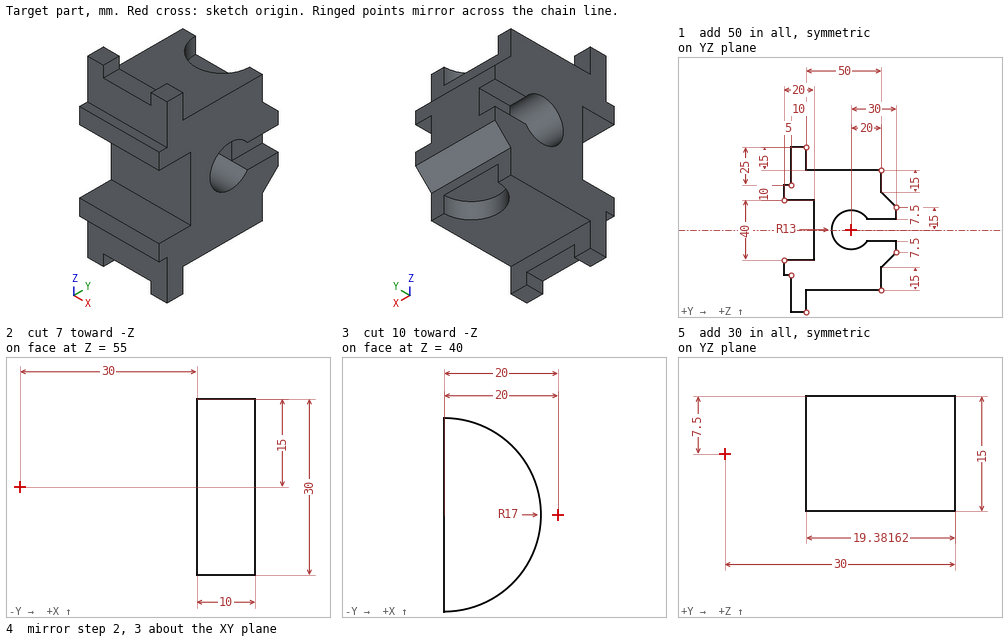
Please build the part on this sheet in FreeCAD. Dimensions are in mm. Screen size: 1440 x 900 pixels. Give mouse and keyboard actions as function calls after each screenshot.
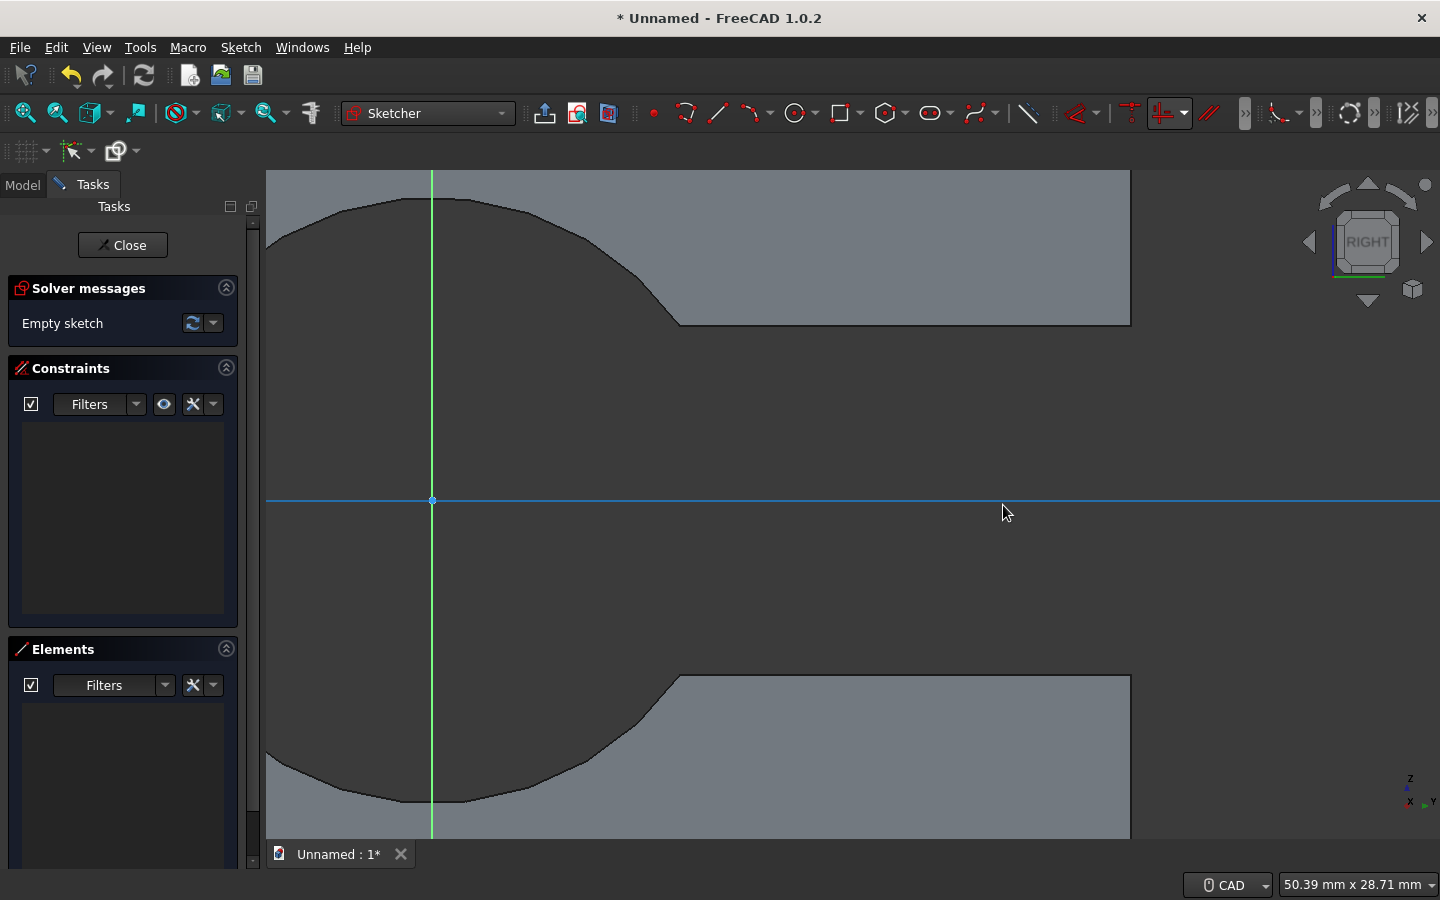
click(840, 114)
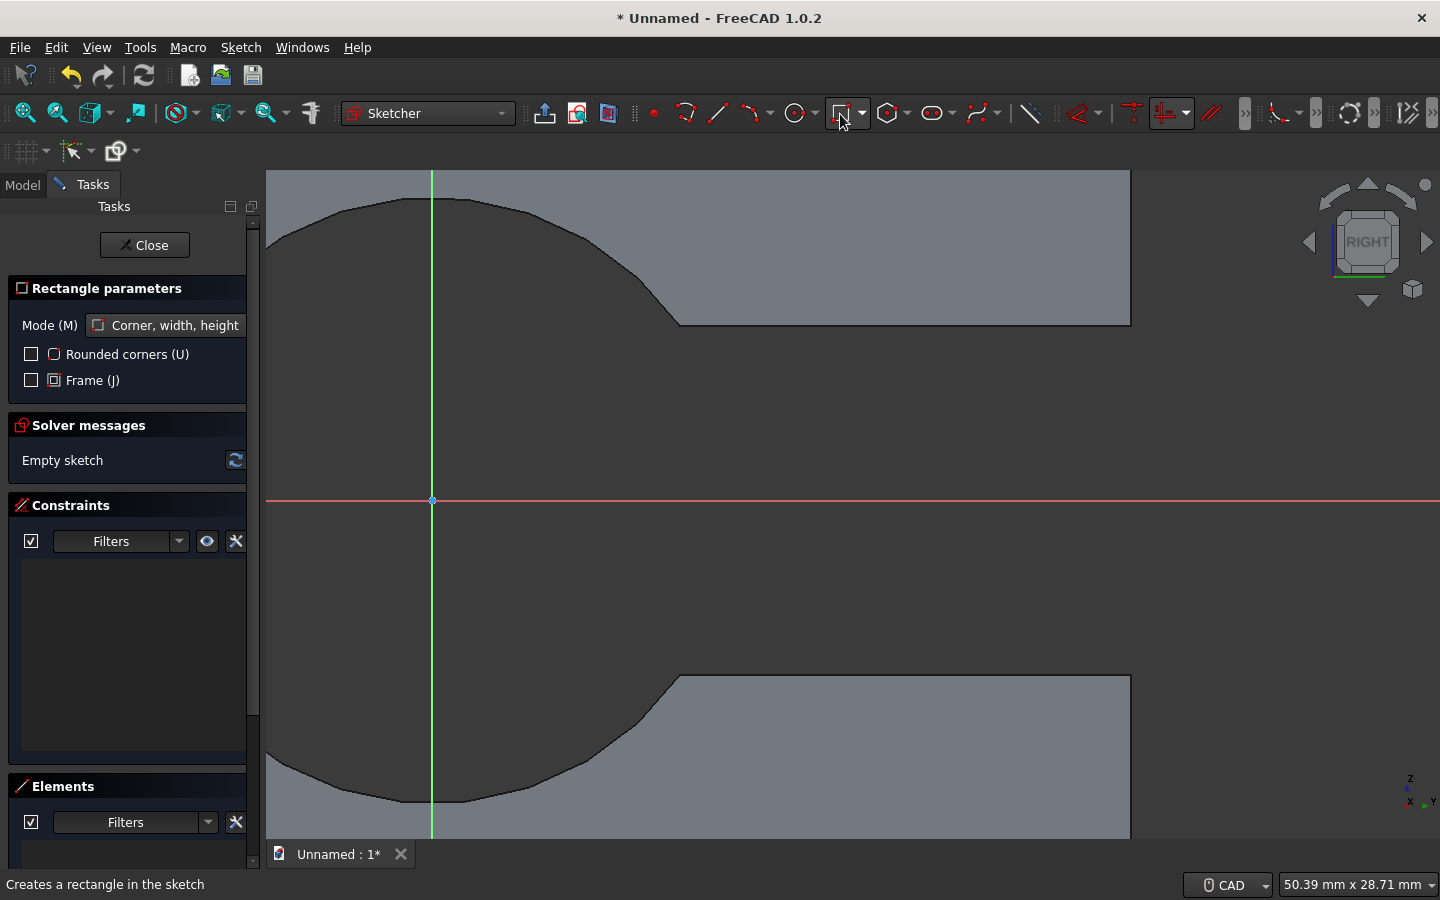
click(680, 326)
move(1131, 675)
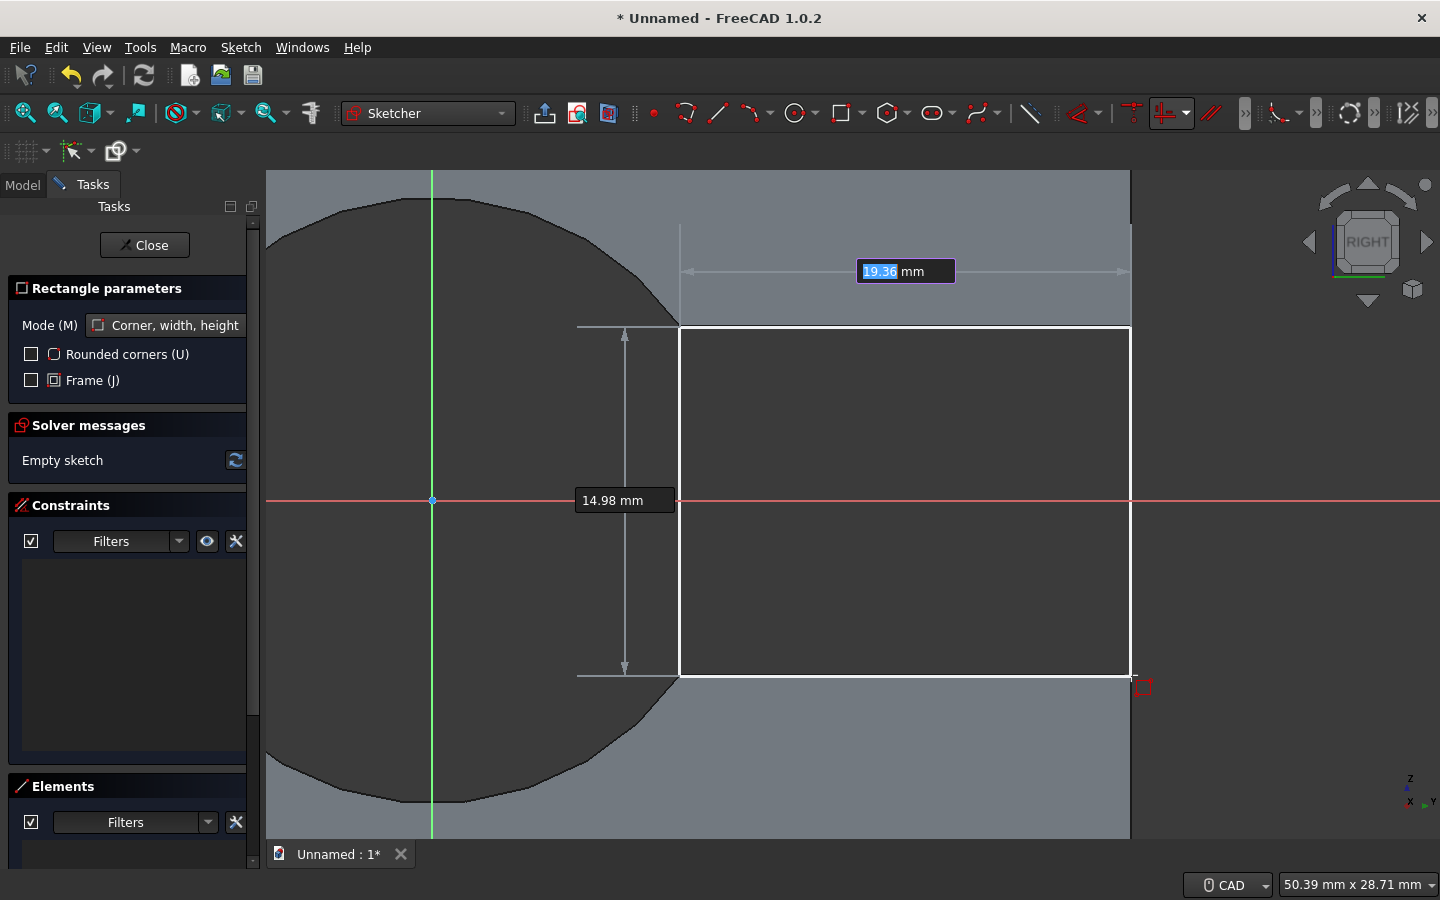
text(19.38162)
key(Tab)
text(15)
key(Return)
key(Escape)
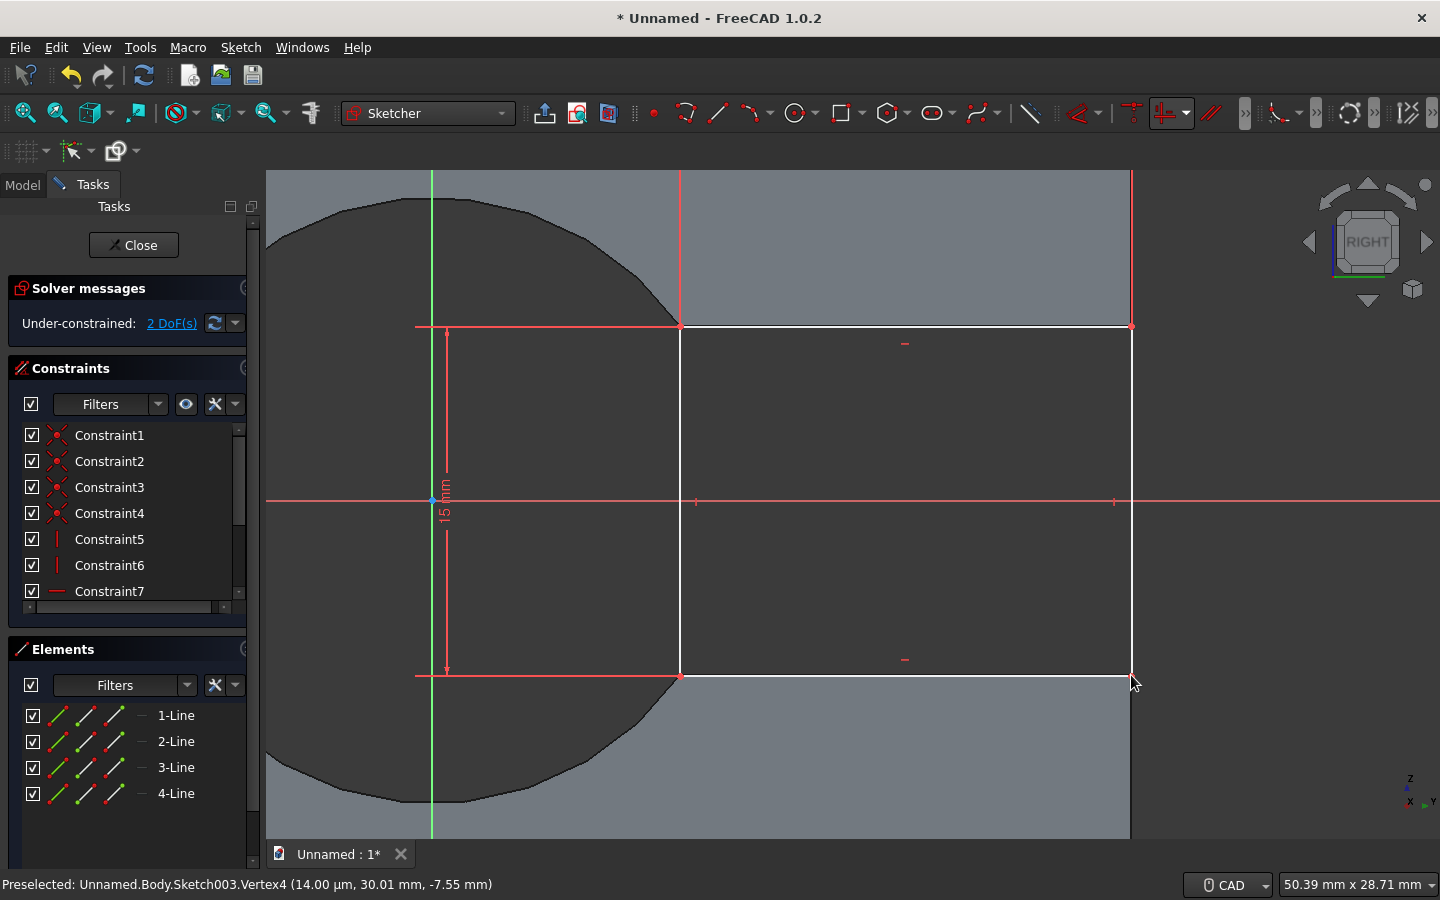
click(1078, 114)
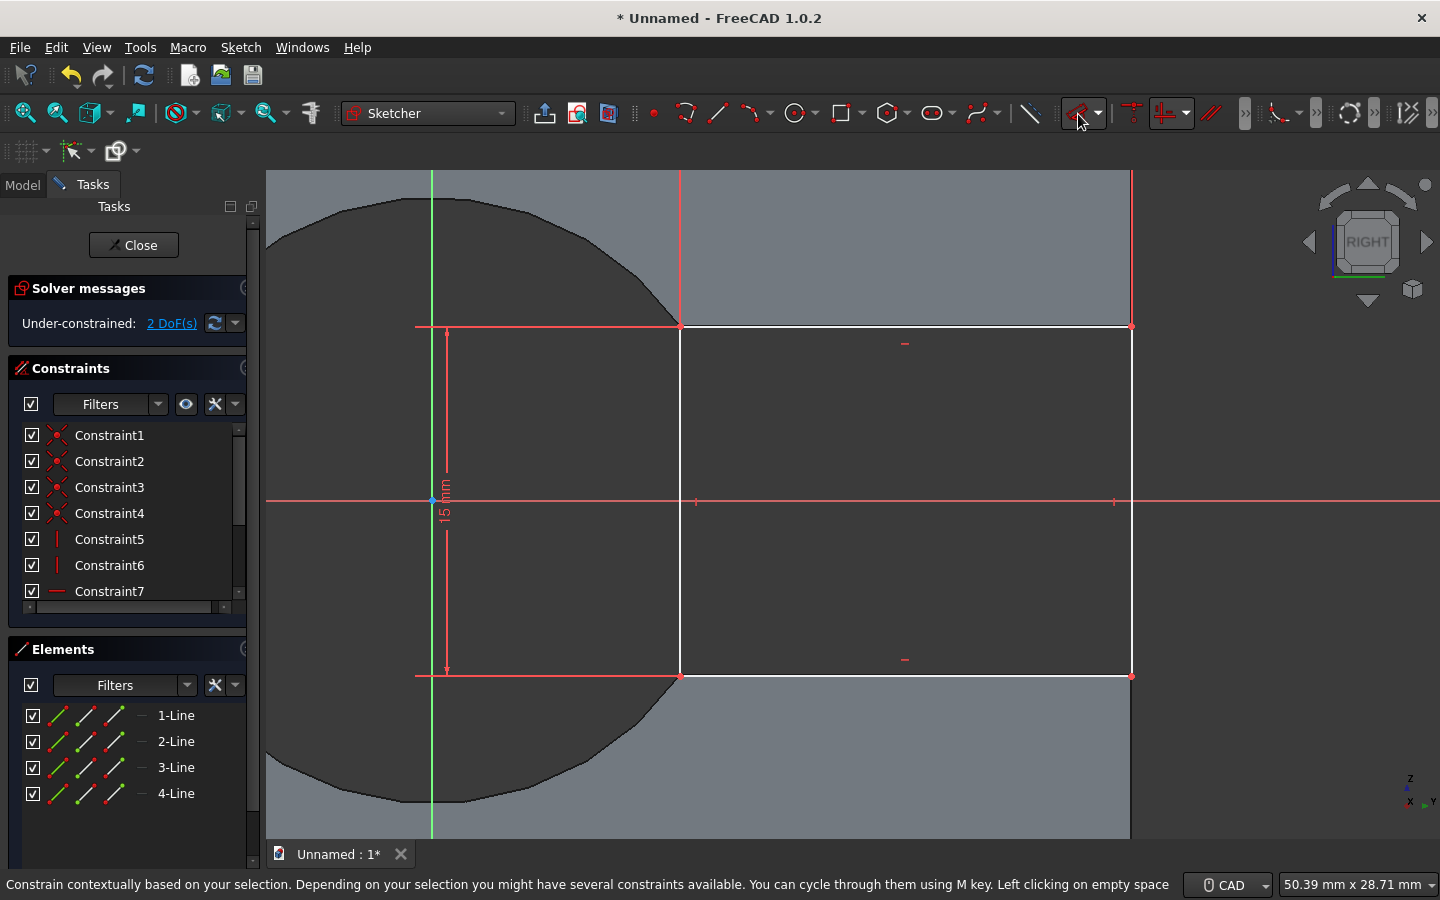
click(1132, 676)
click(782, 710)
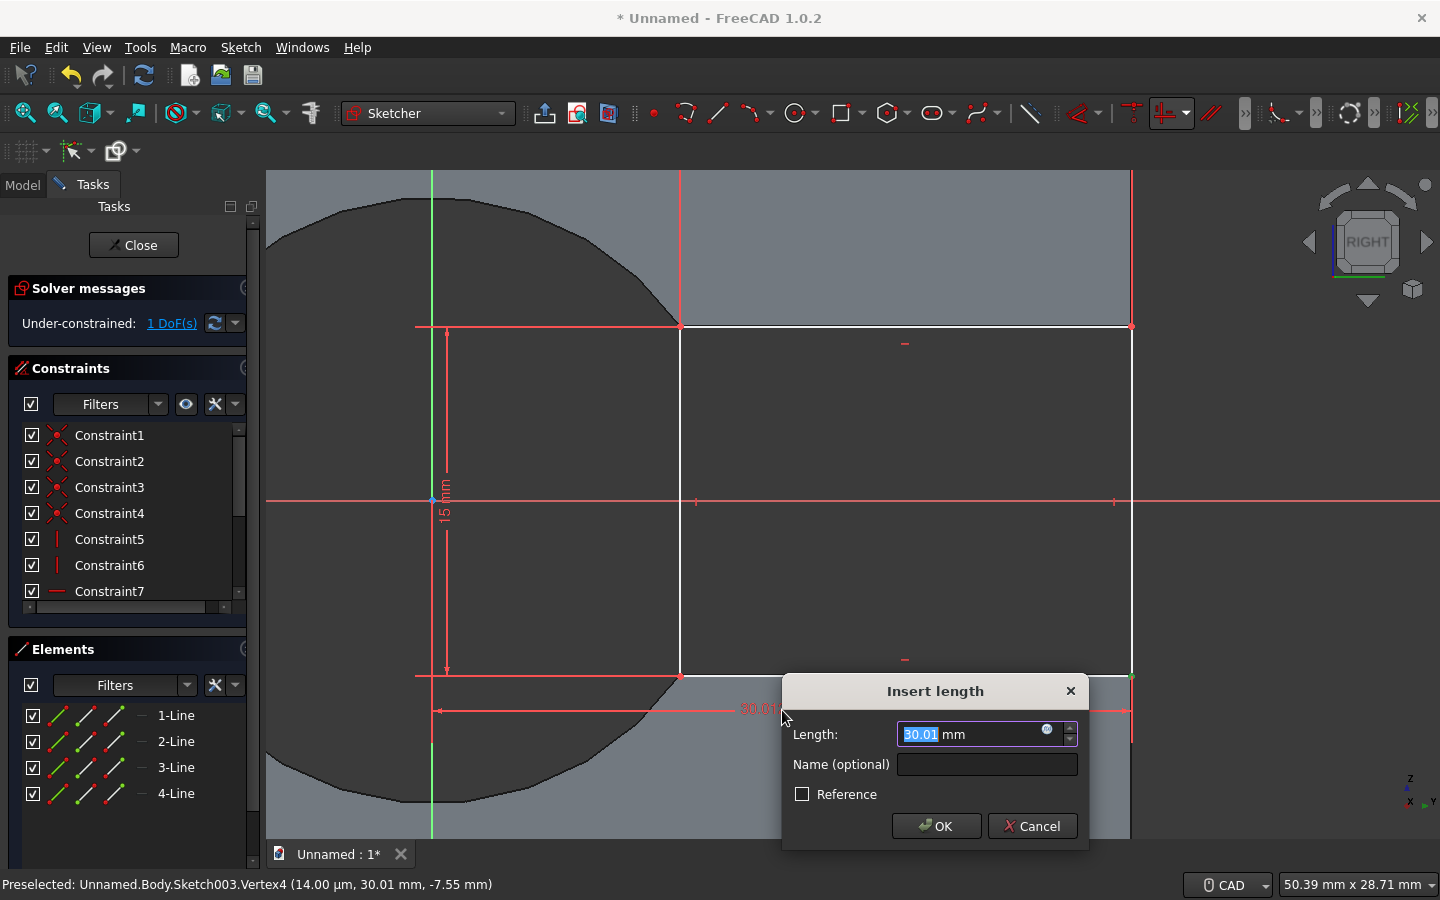
text(30)
key(Return)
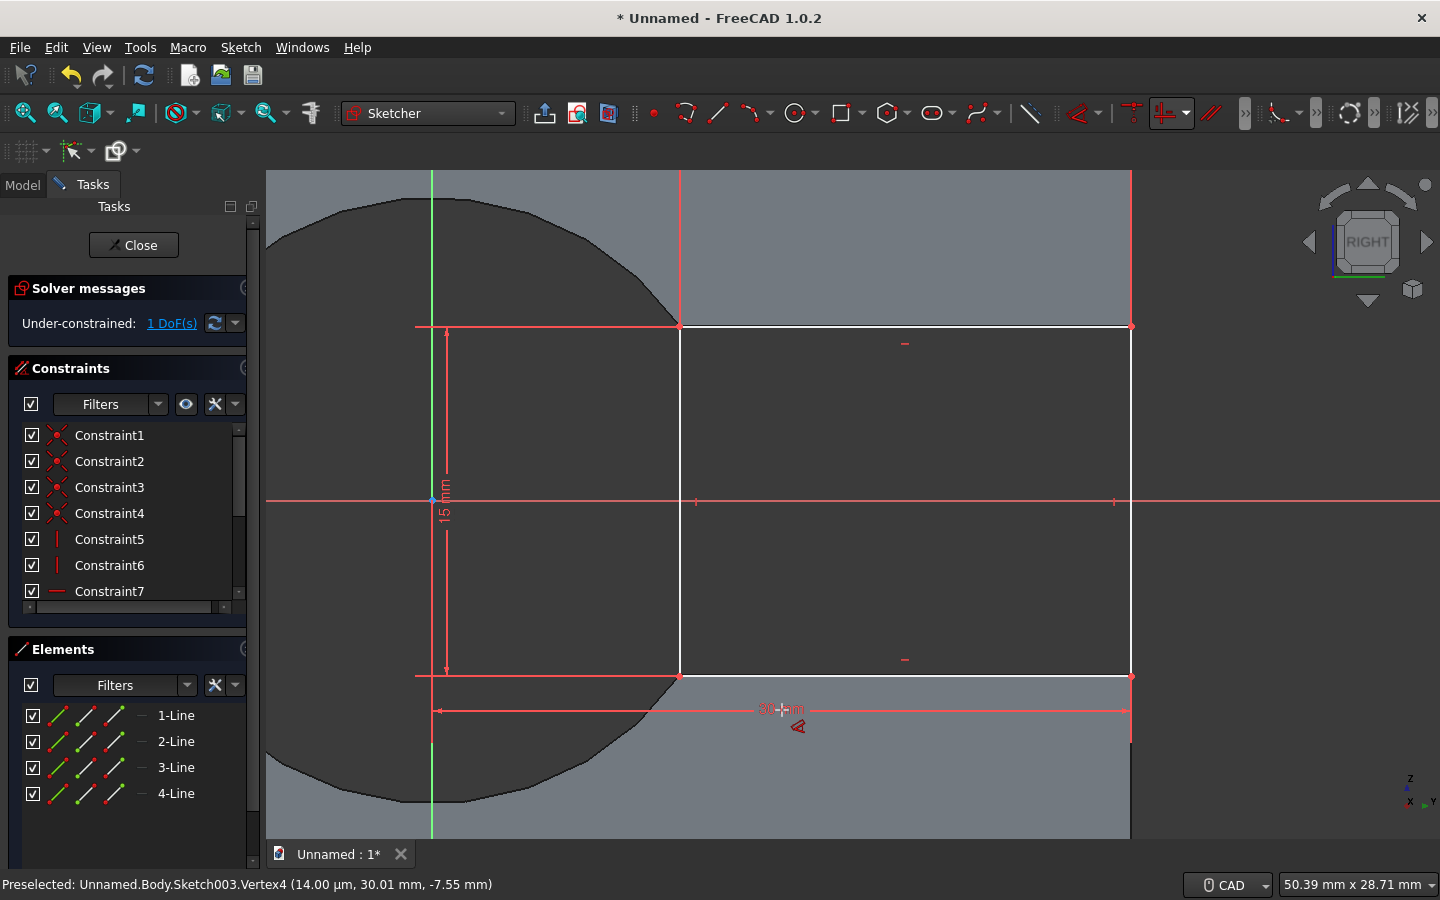
click(680, 327)
click(398, 414)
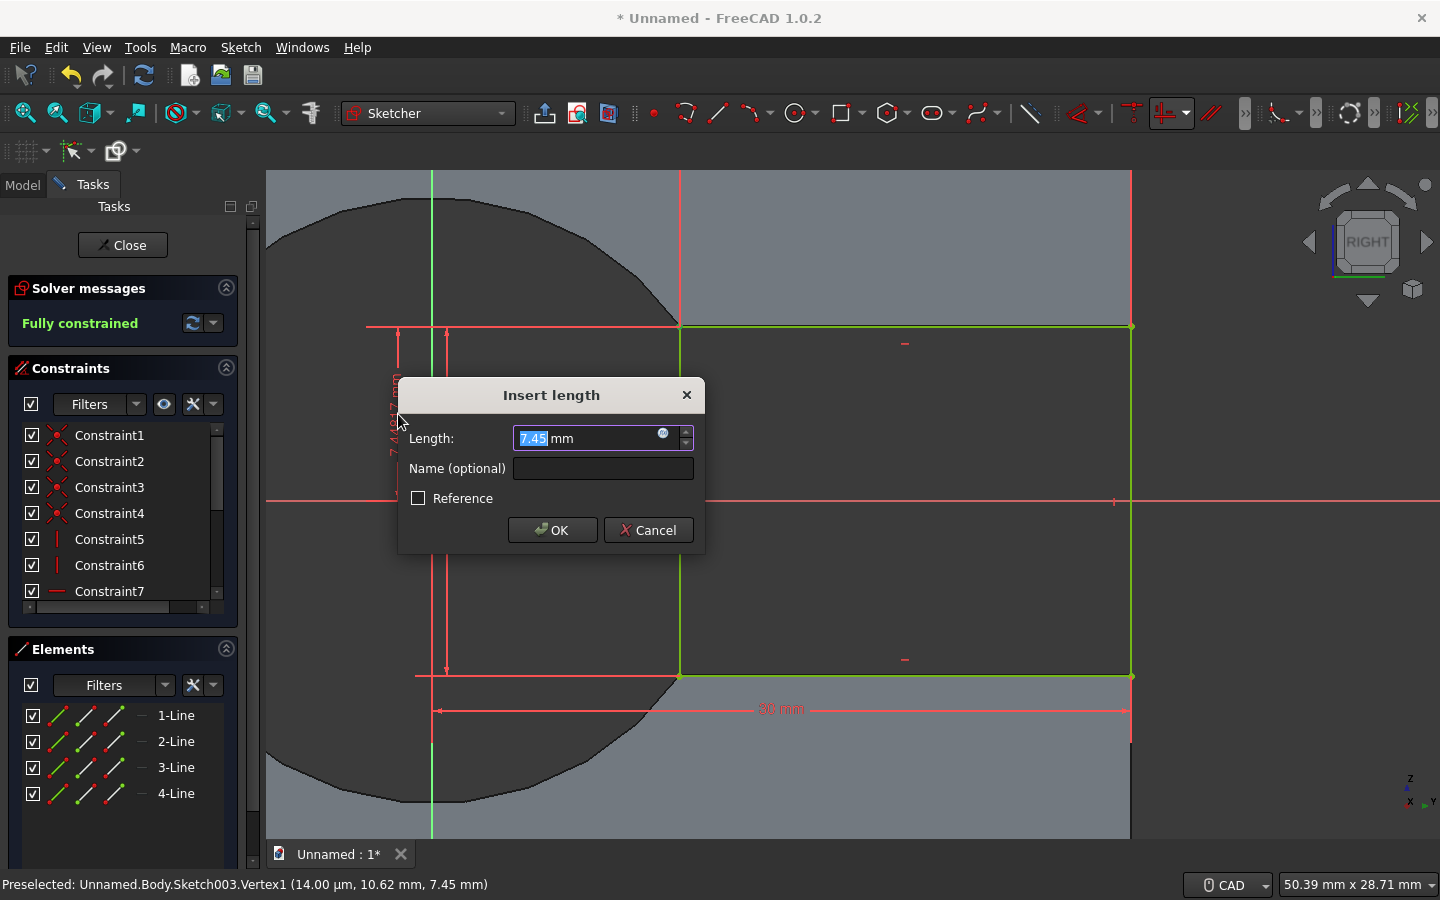
text(7.5)
key(Return)
key(Escape)